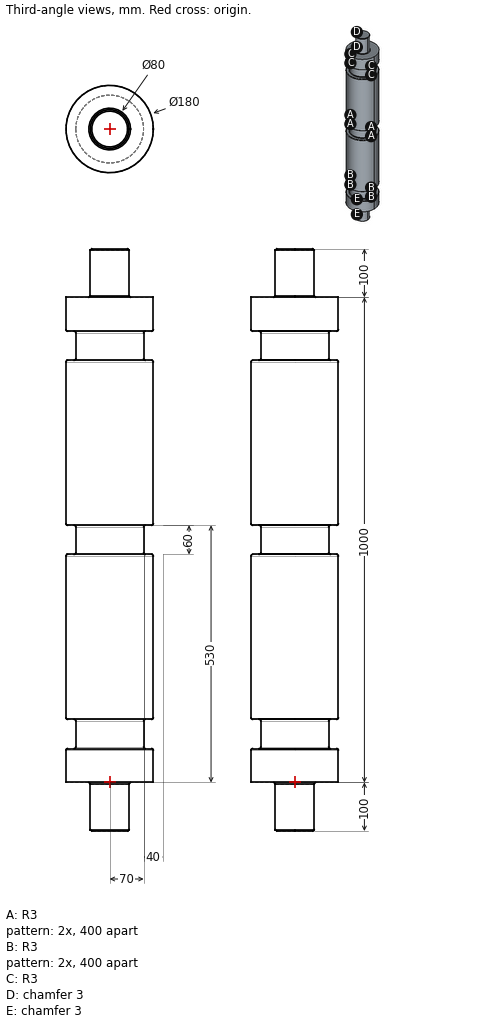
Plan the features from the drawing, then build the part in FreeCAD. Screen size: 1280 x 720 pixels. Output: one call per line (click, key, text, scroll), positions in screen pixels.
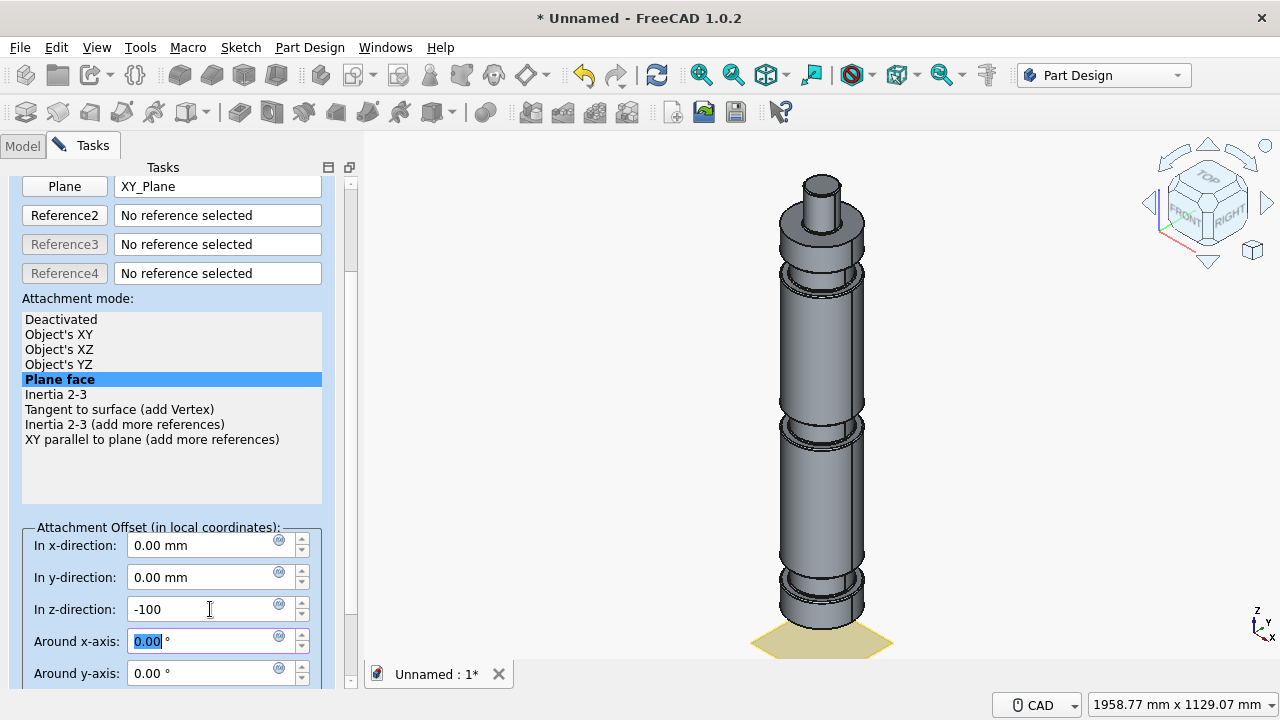
scroll(351, 432, up, 3)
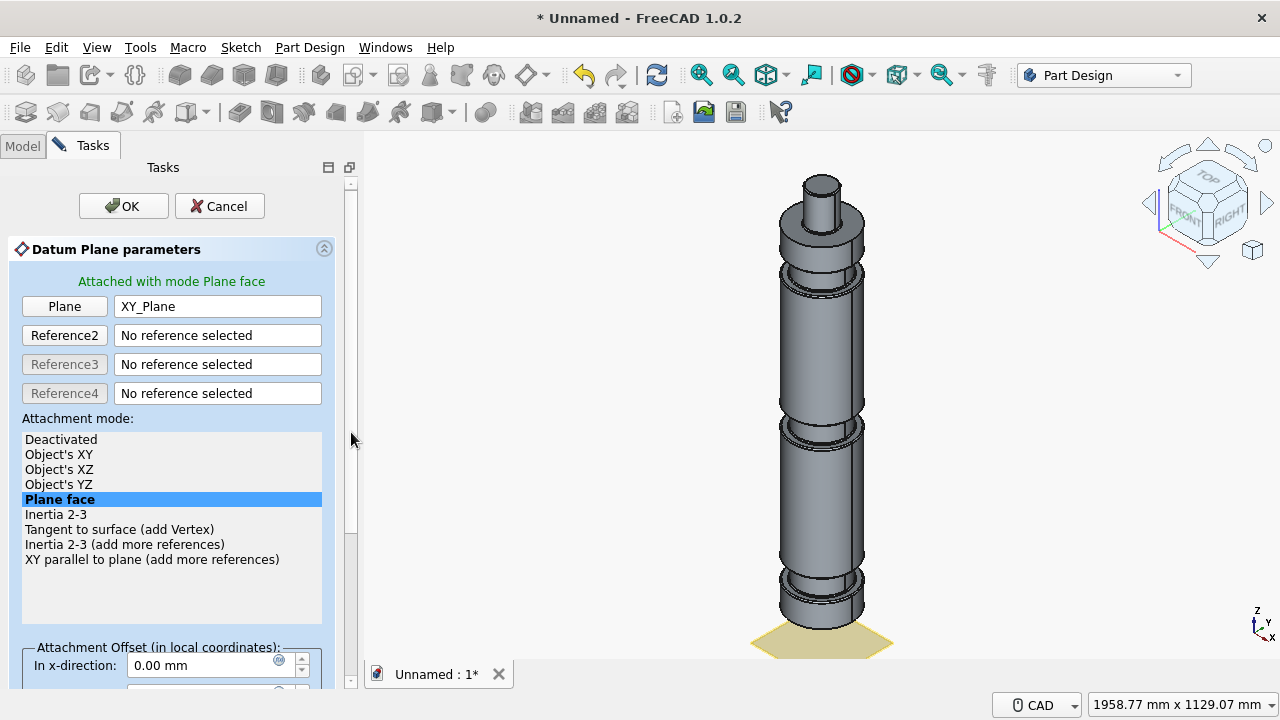
click(124, 206)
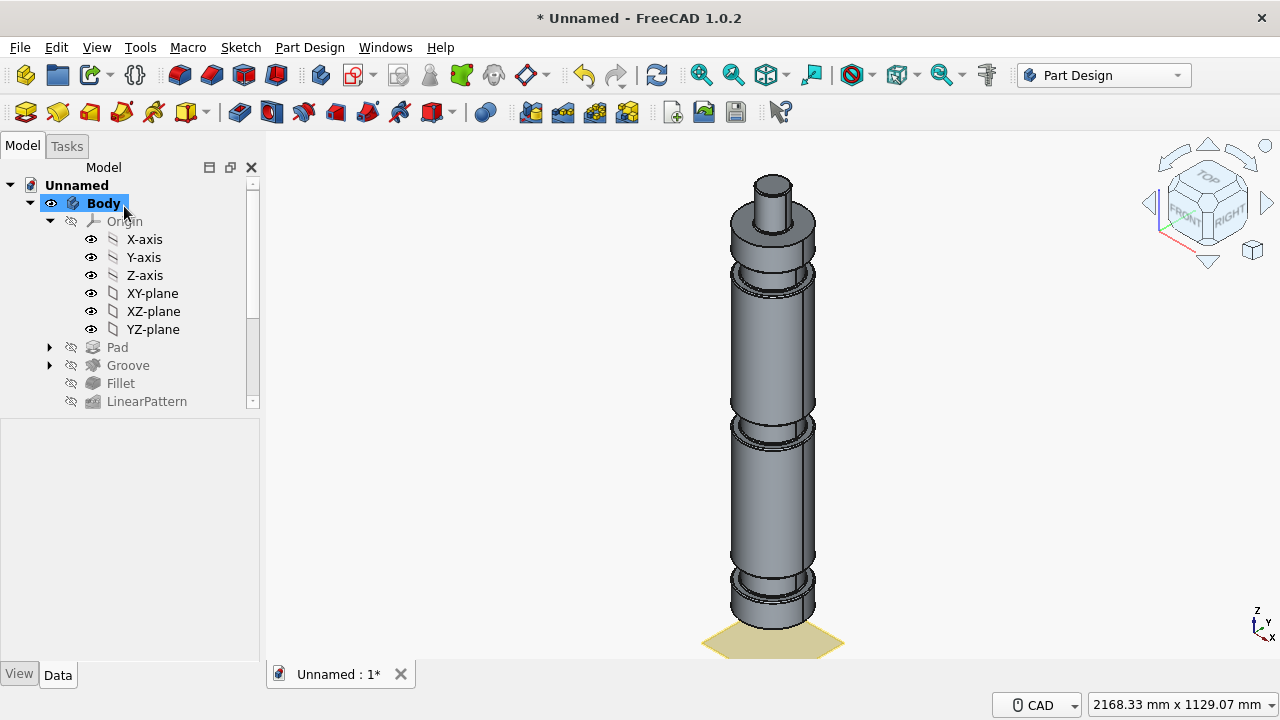
scroll(100, 289, down, 3)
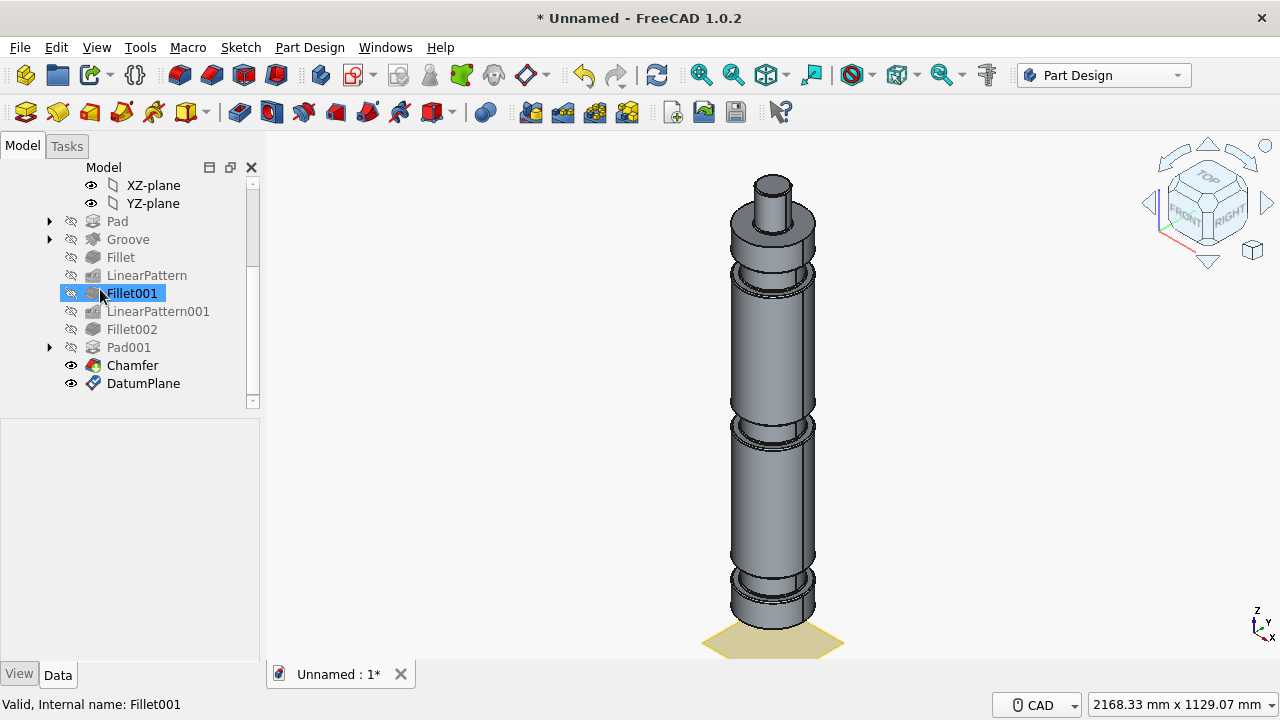
click(116, 383)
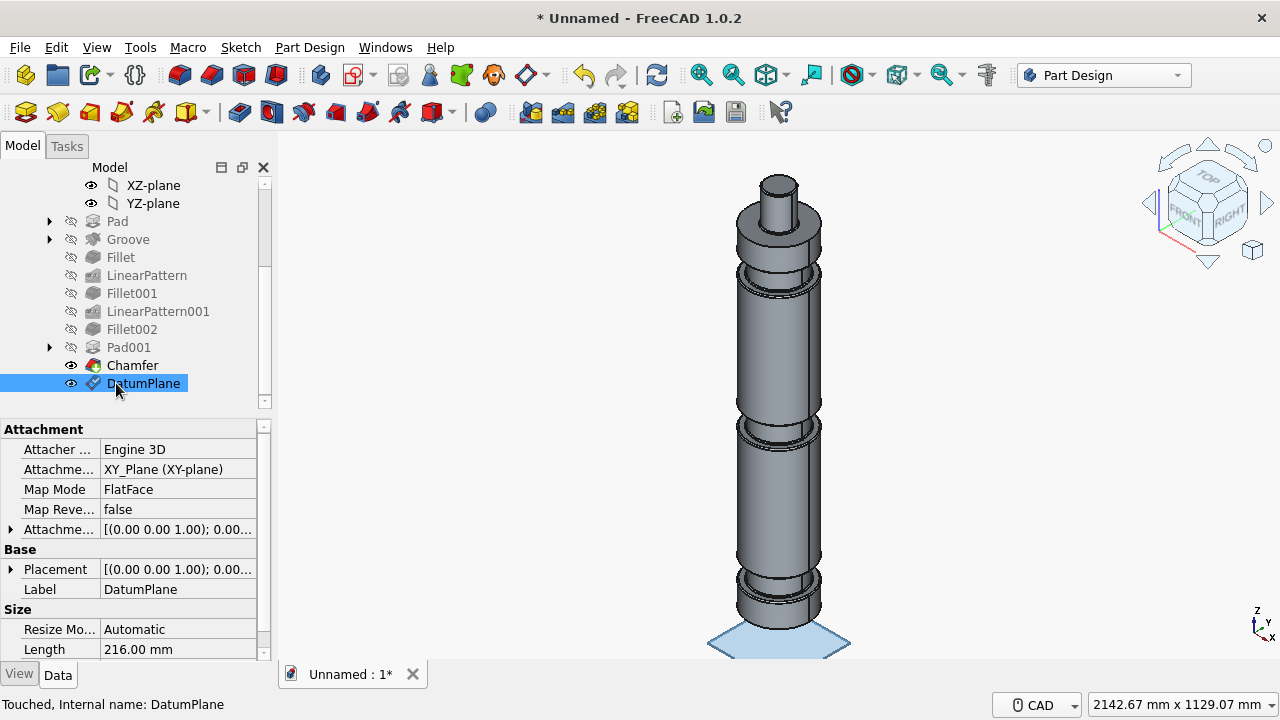
click(354, 76)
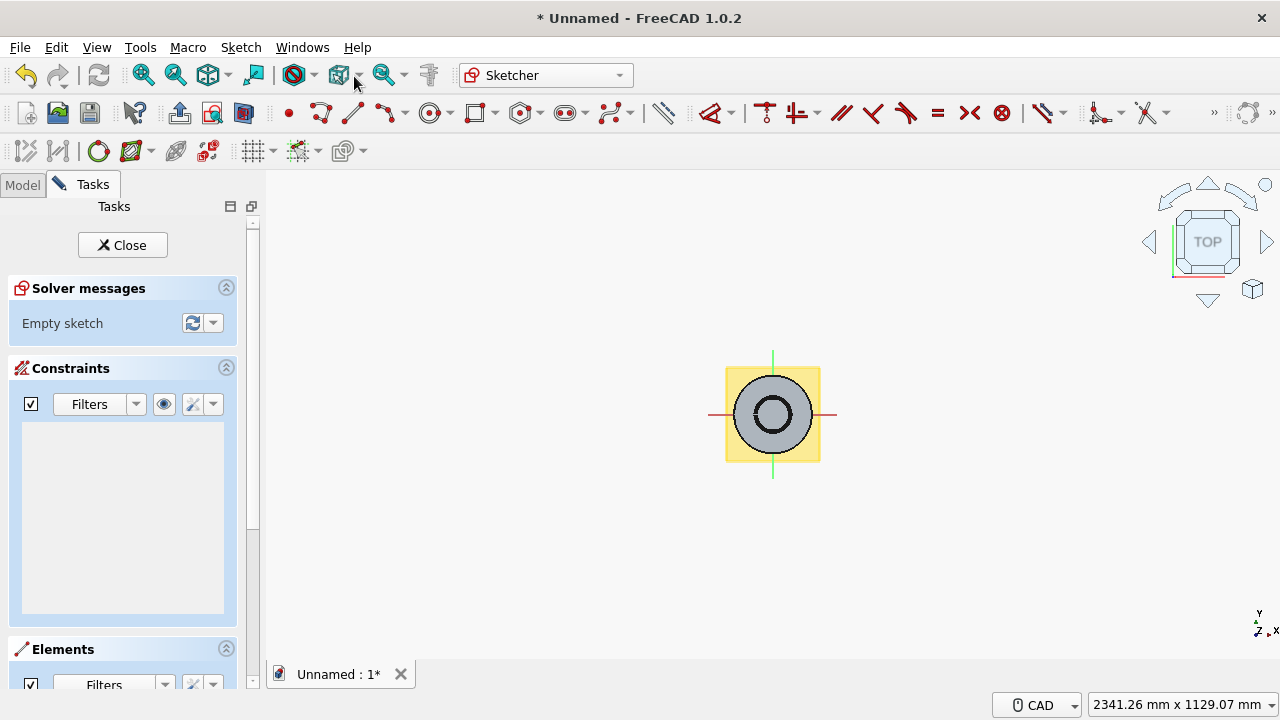
click(244, 114)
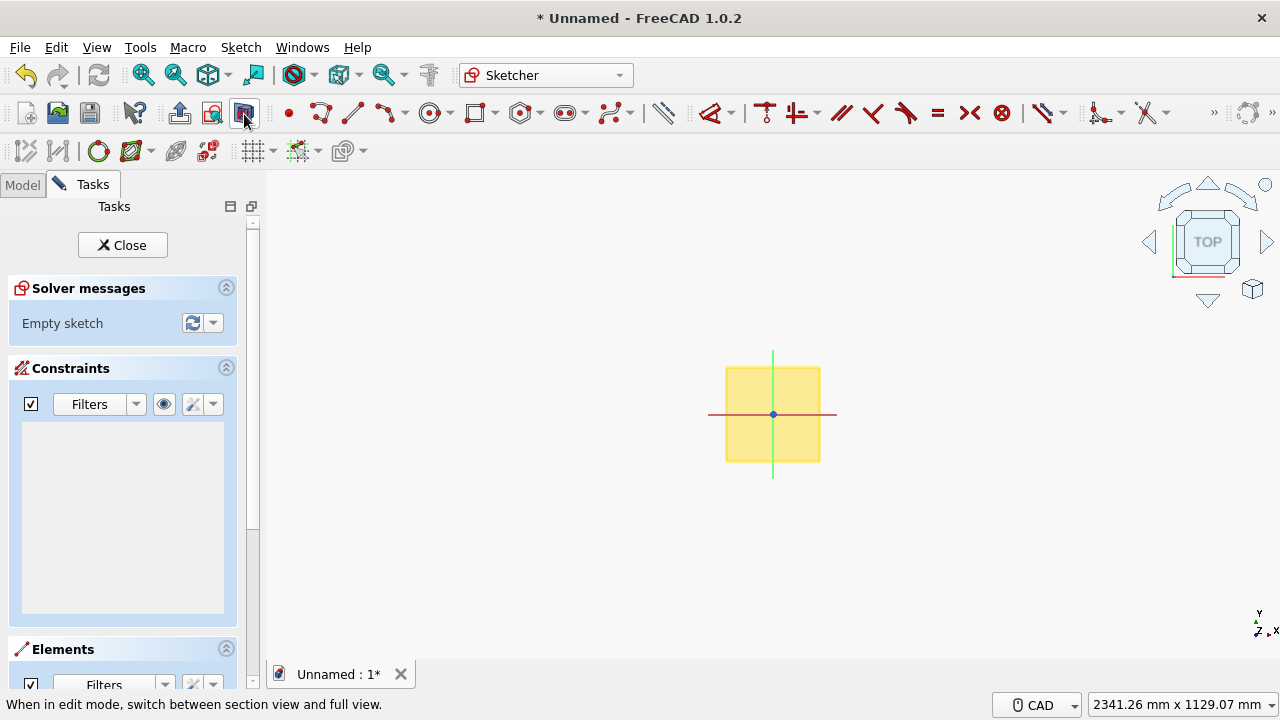
scroll(782, 414, up, 11)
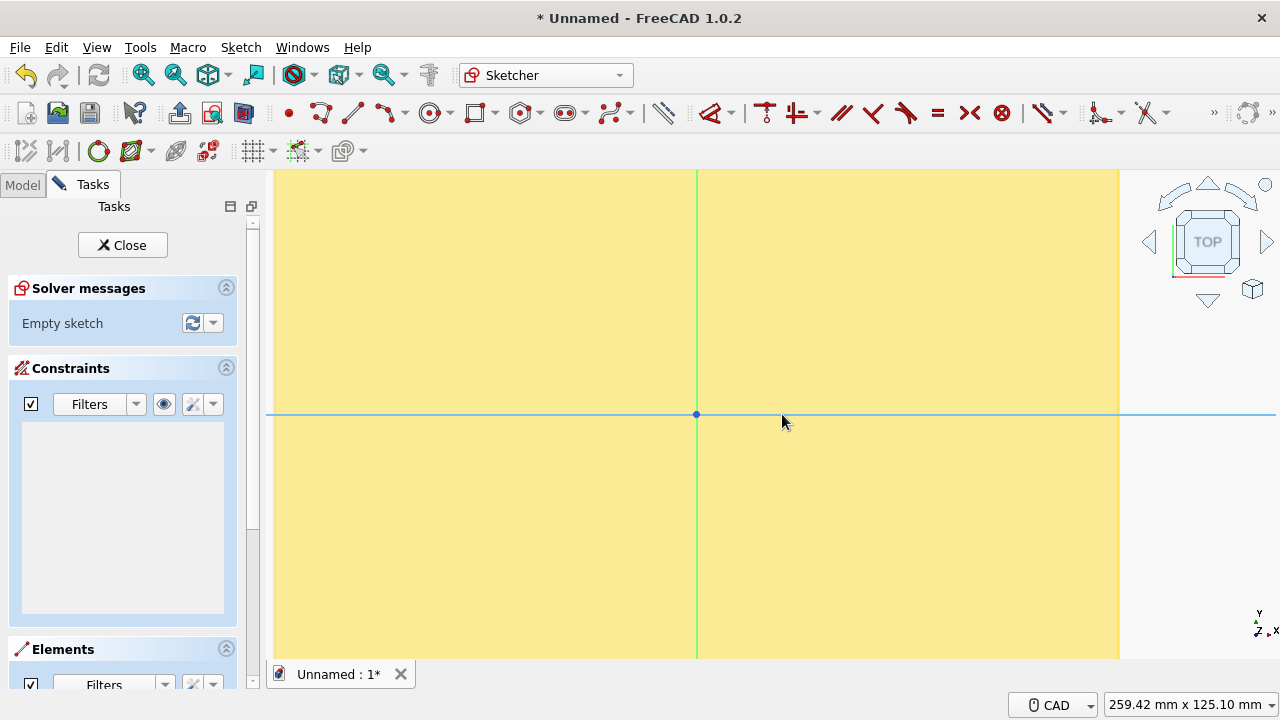
click(430, 114)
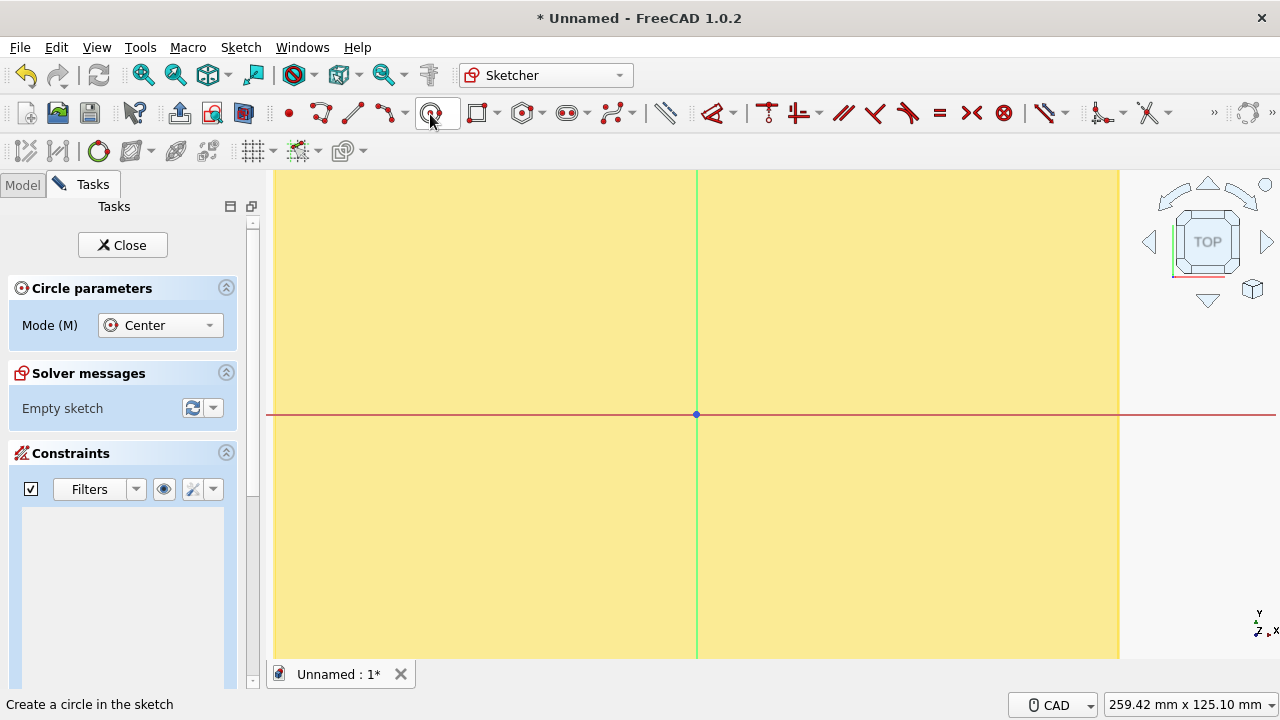
click(697, 414)
move(807, 304)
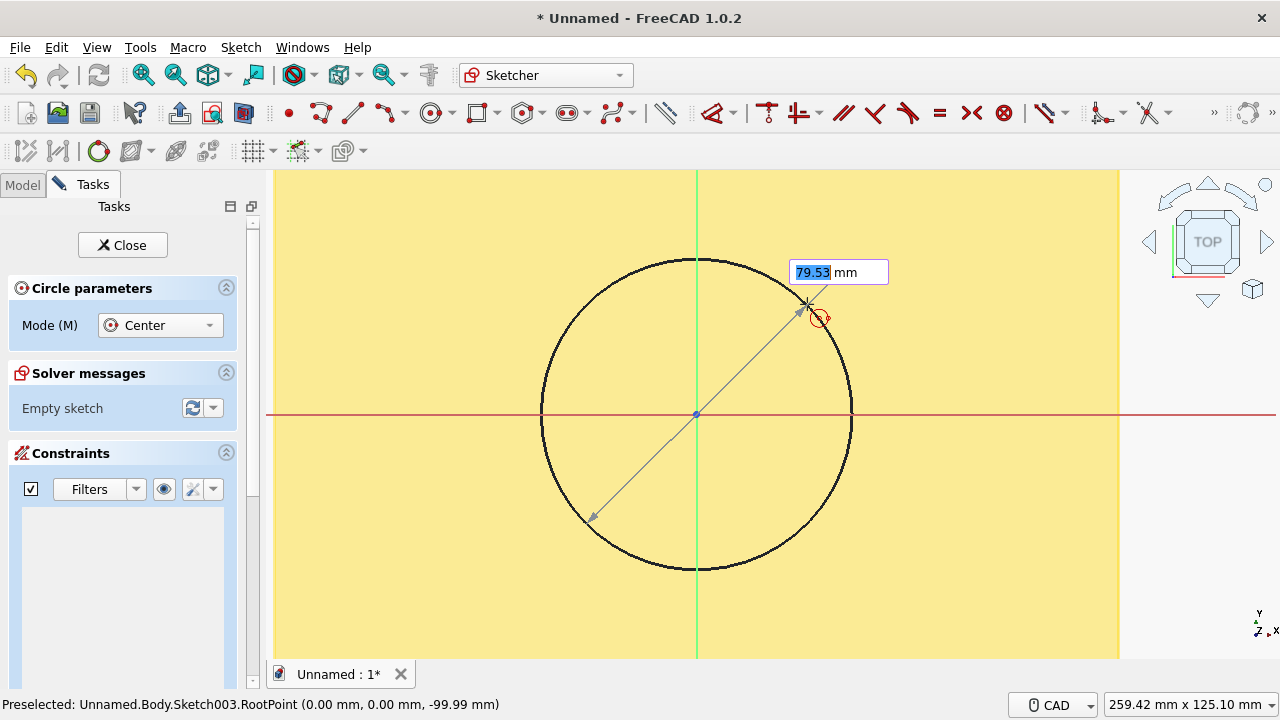
text(80)
key(Return)
key(Escape)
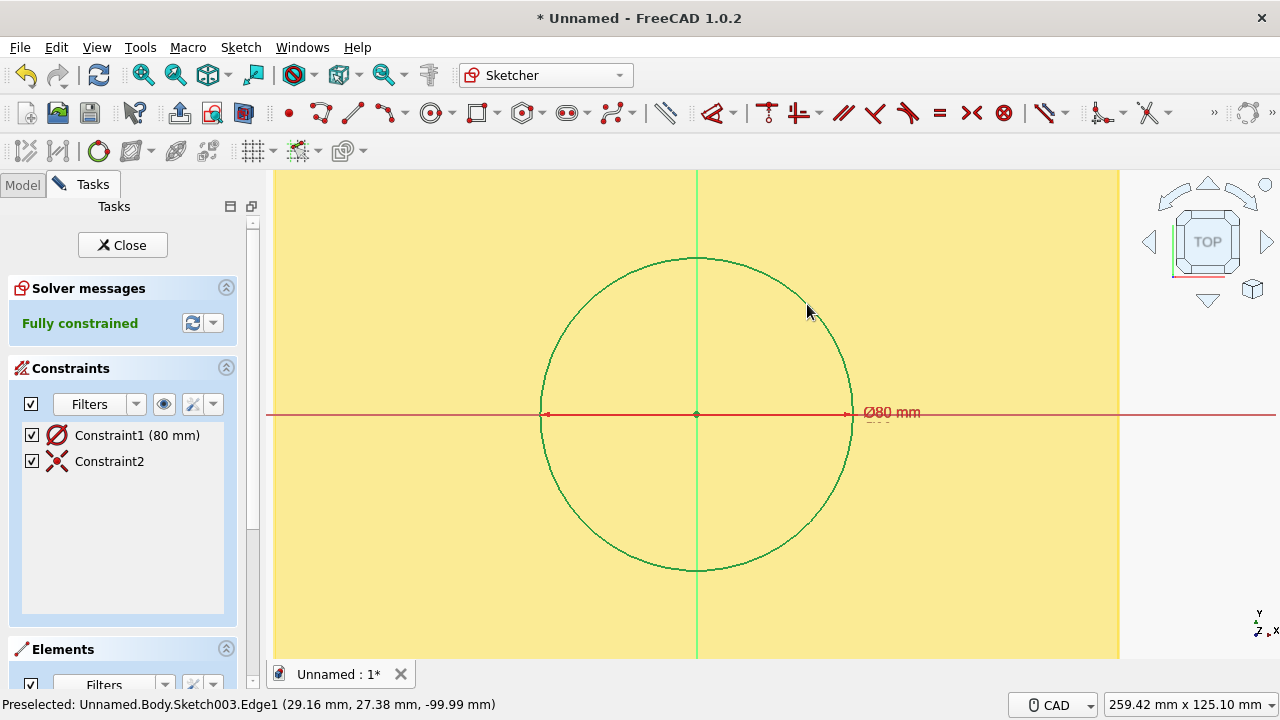
click(123, 245)